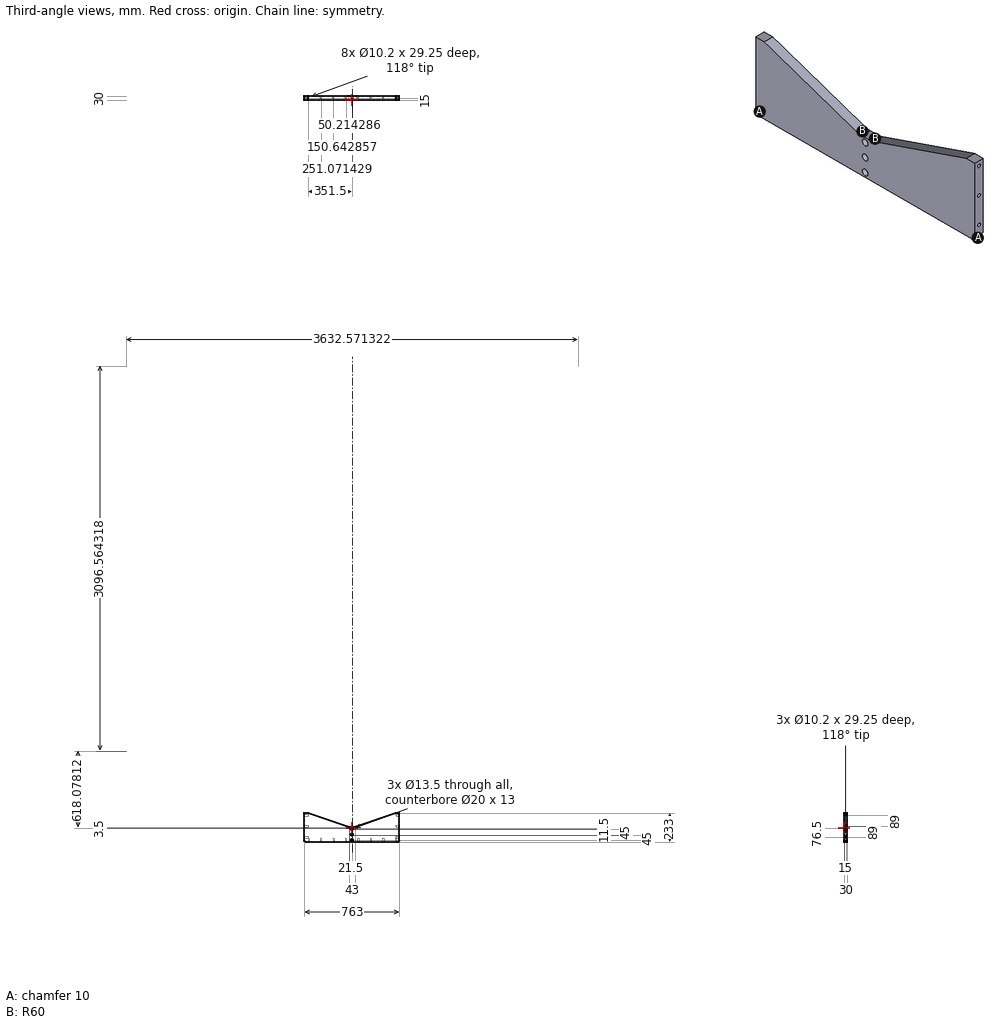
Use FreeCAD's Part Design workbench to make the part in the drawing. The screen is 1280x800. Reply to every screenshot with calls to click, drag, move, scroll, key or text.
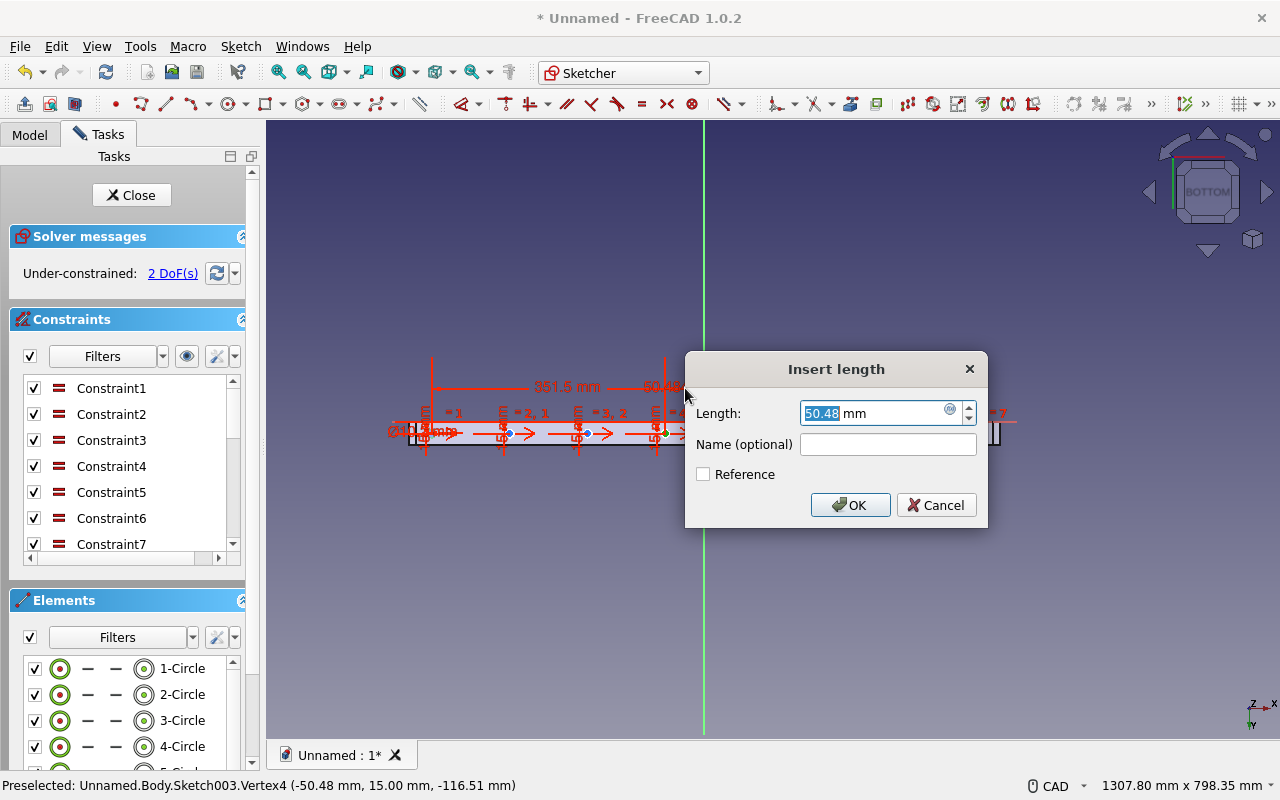
text(50.214286)
key(Return)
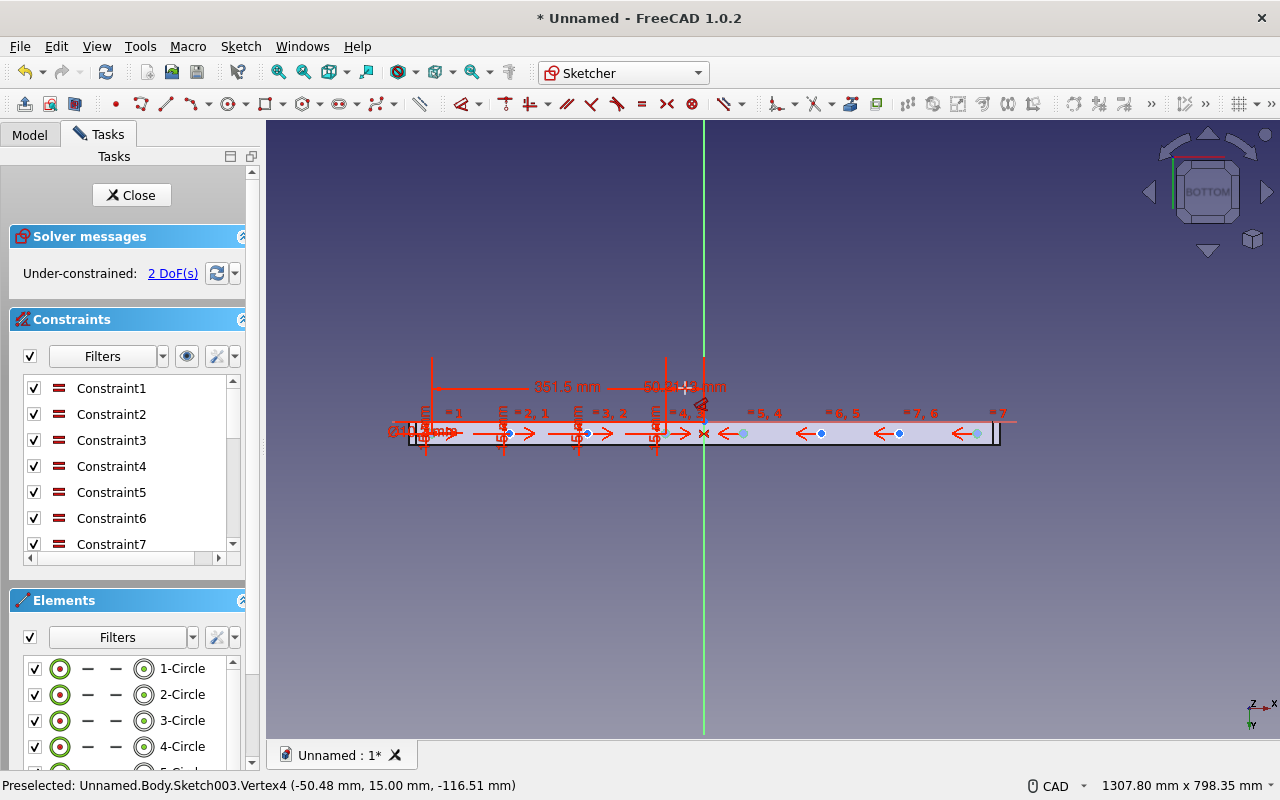
click(510, 434)
click(607, 468)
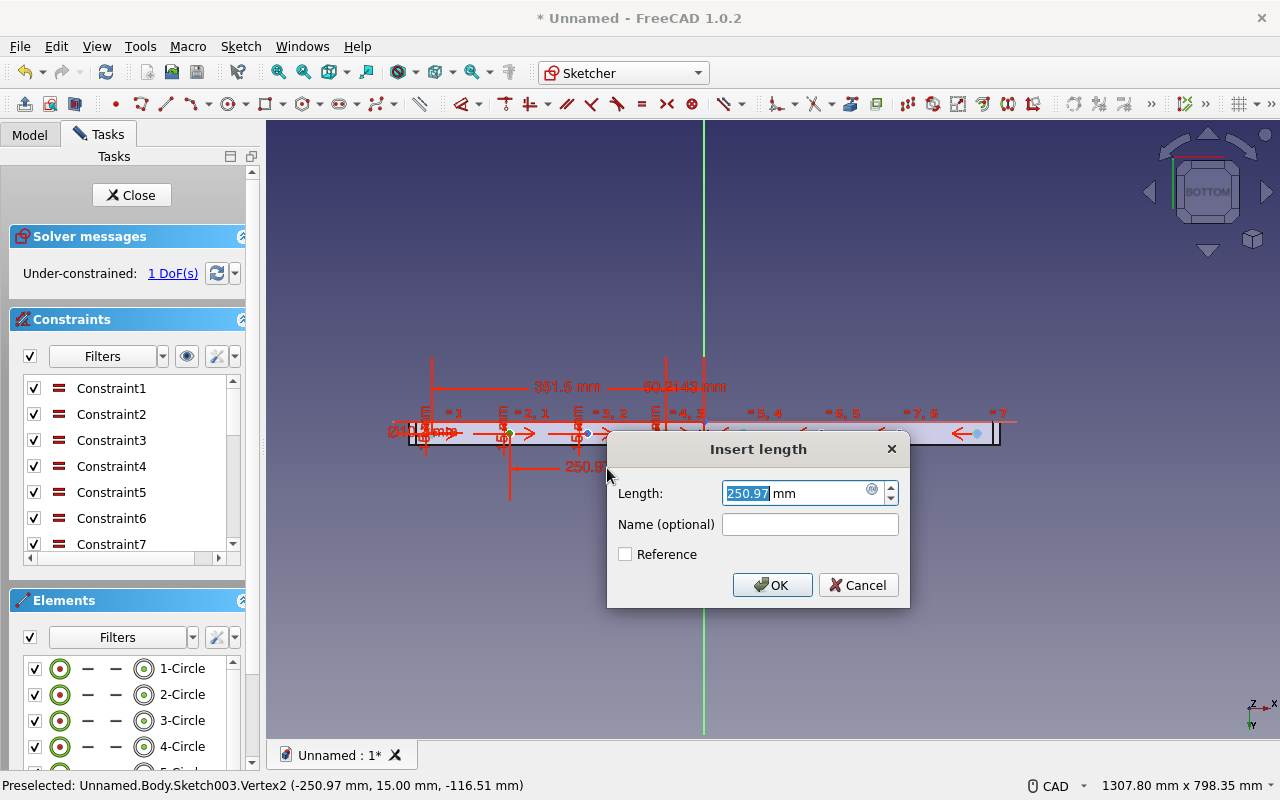
text(251.071429)
key(Return)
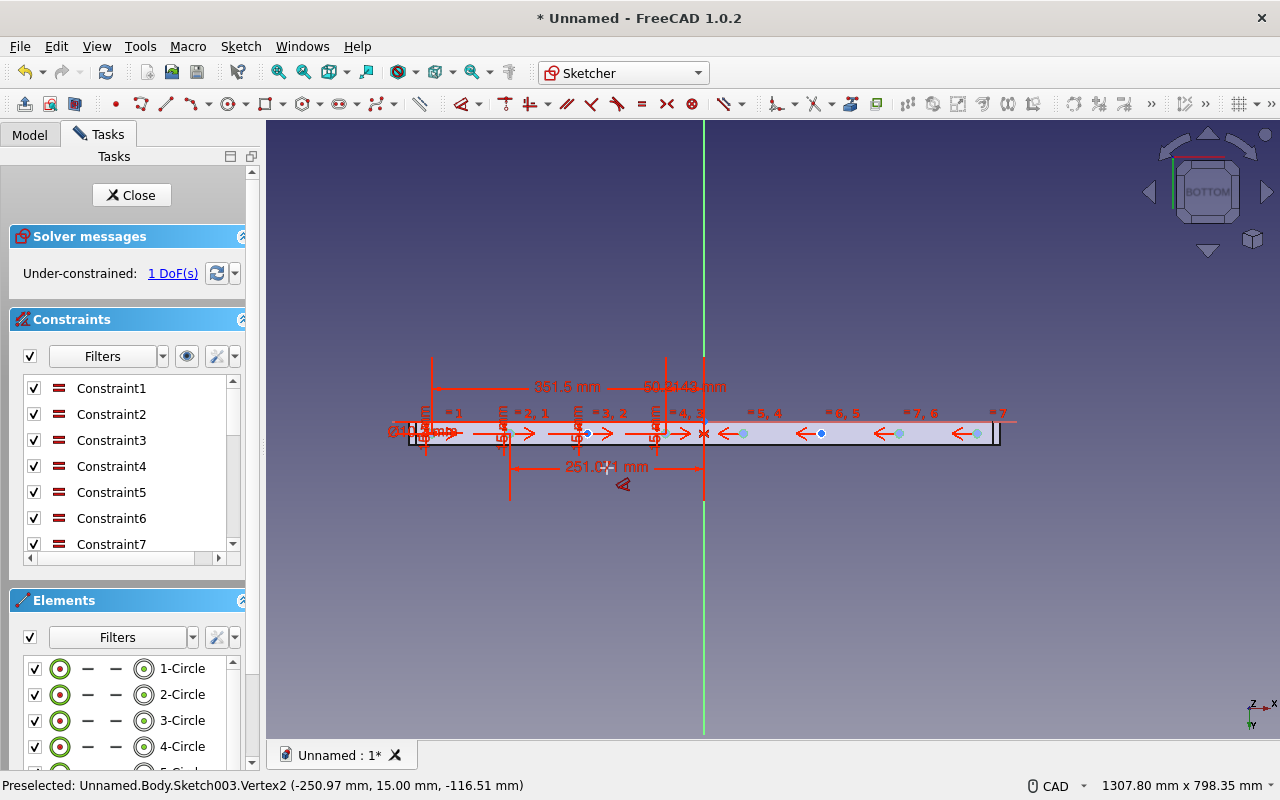
click(588, 434)
click(687, 468)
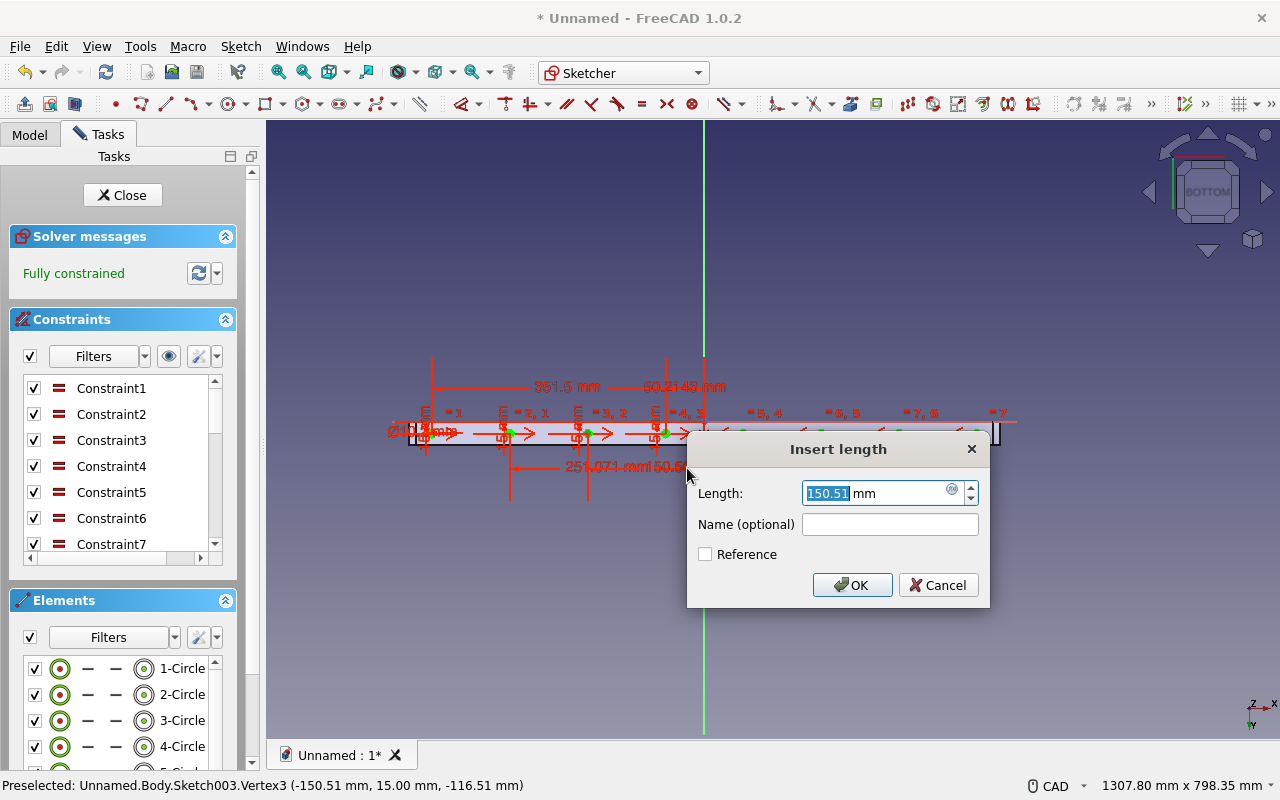
text(150.642857)
key(Return)
key(Escape)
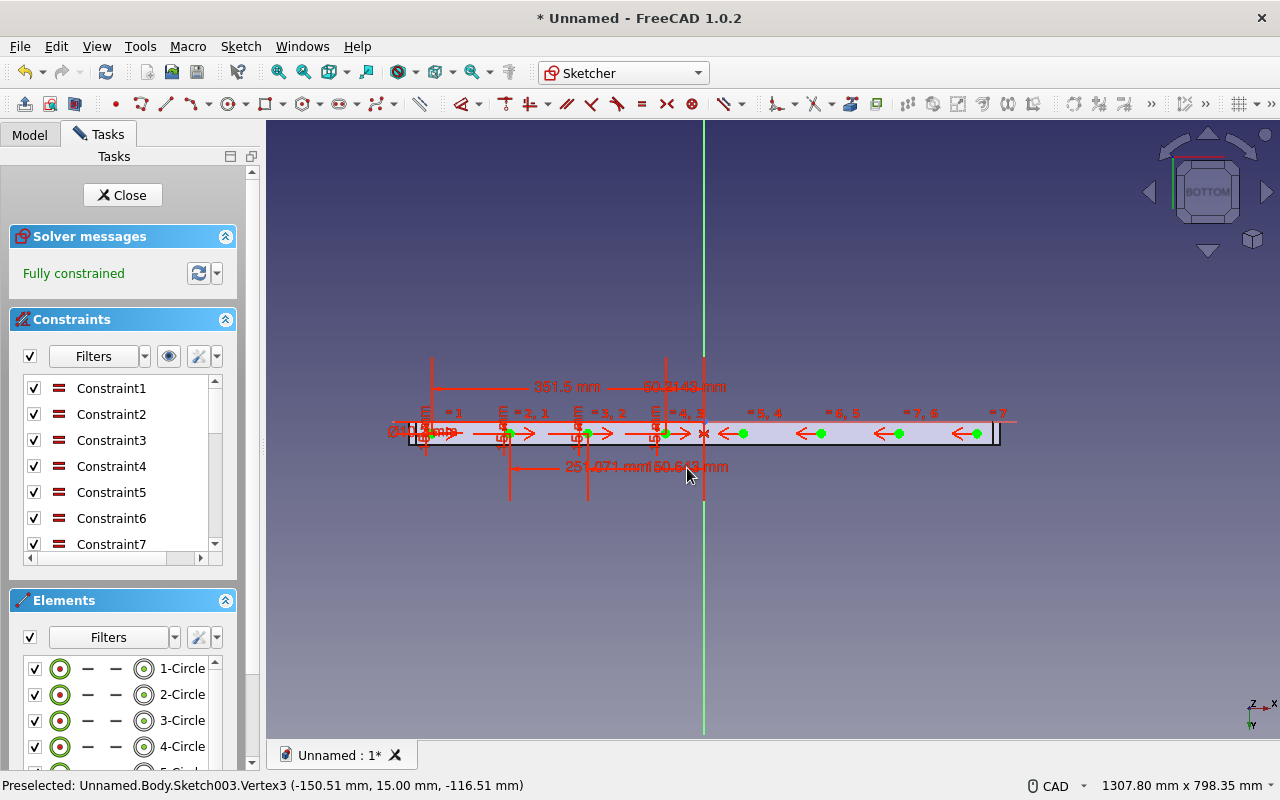
click(123, 195)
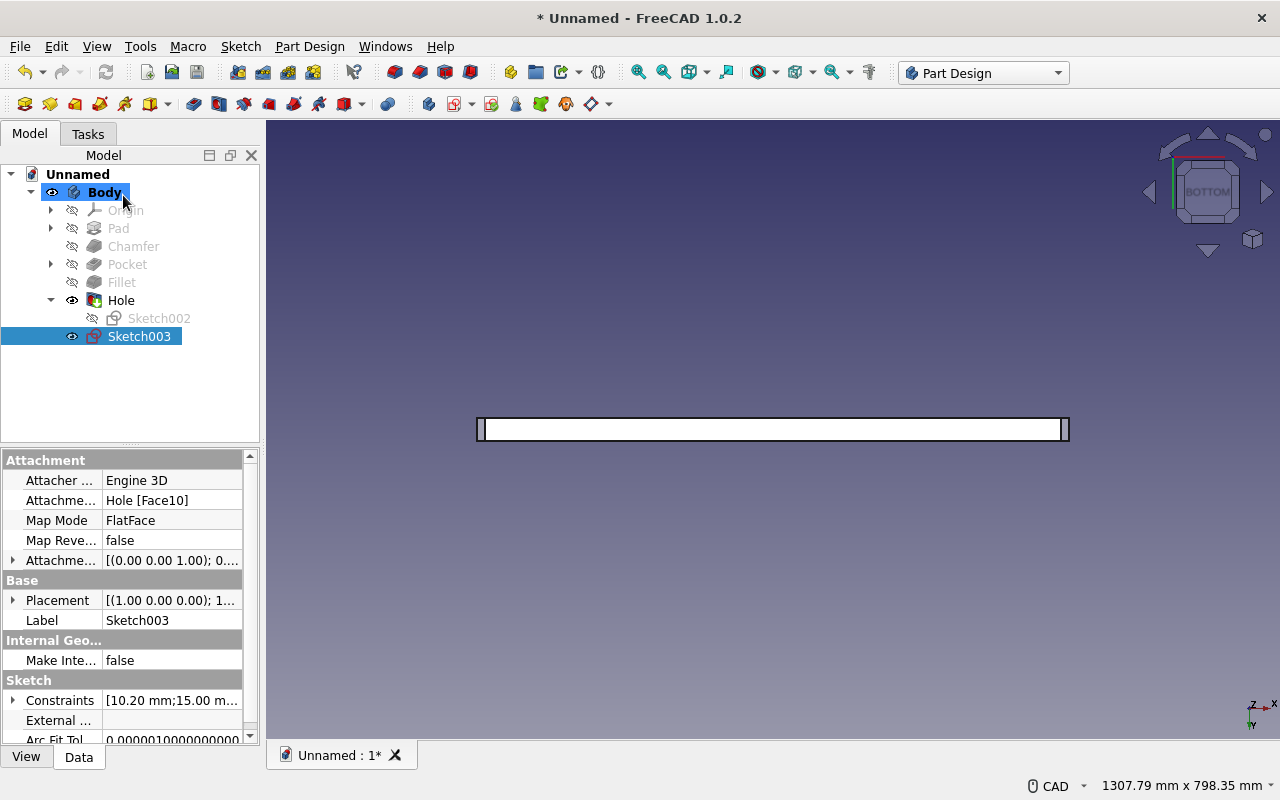
click(219, 104)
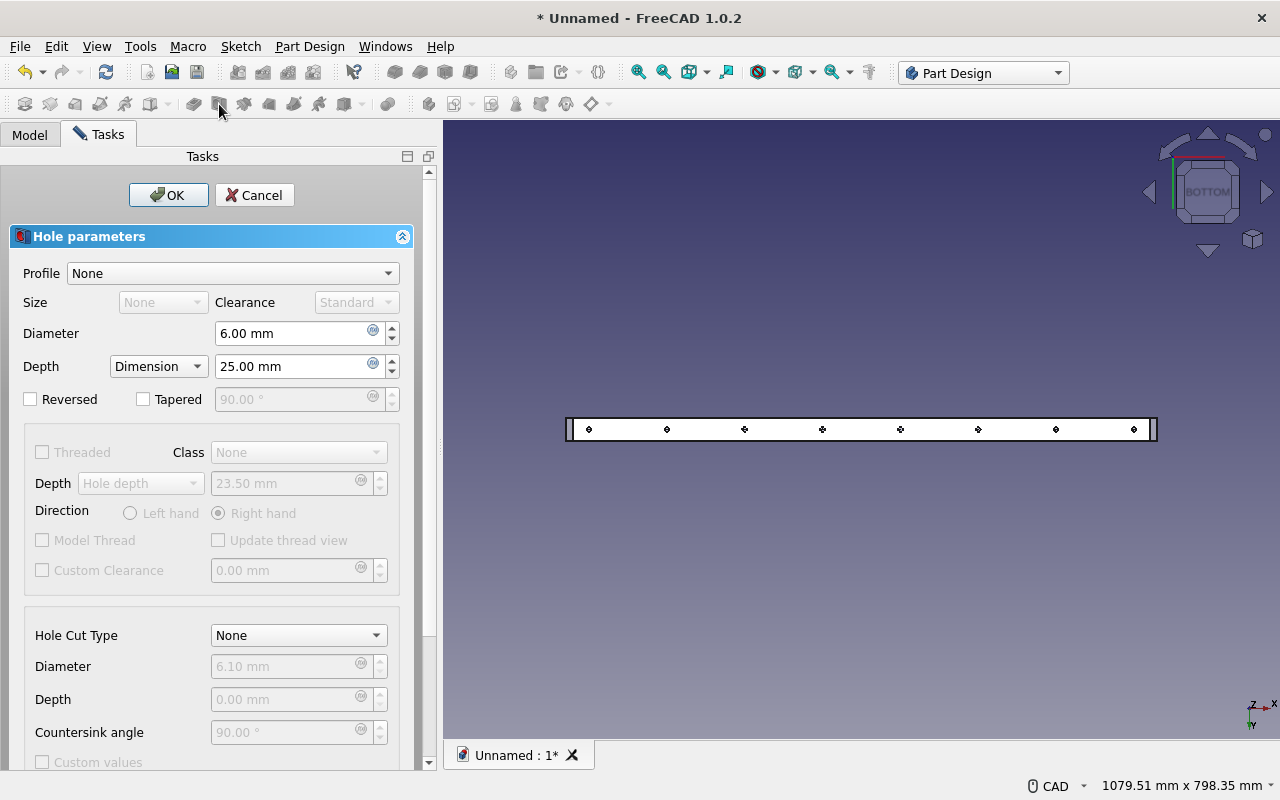
triple_click(300, 334)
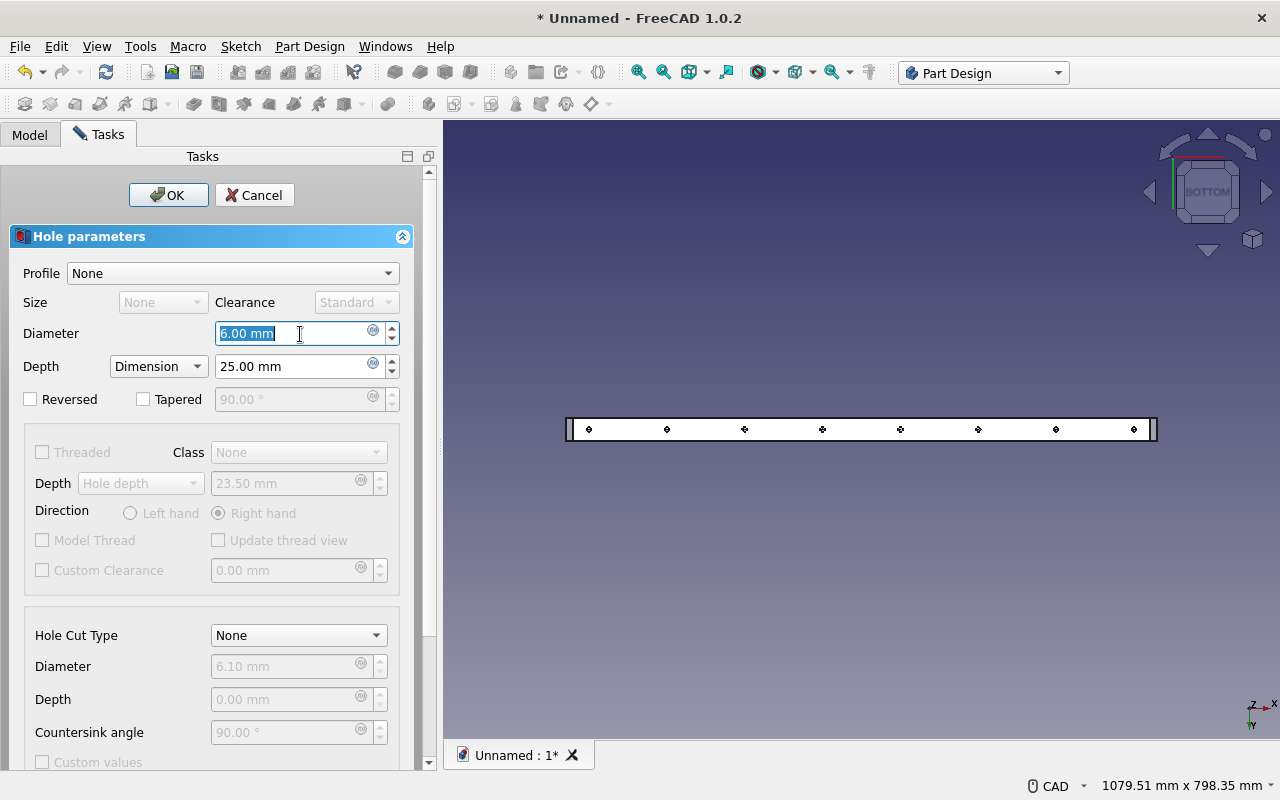
text(10.2)
key(Tab)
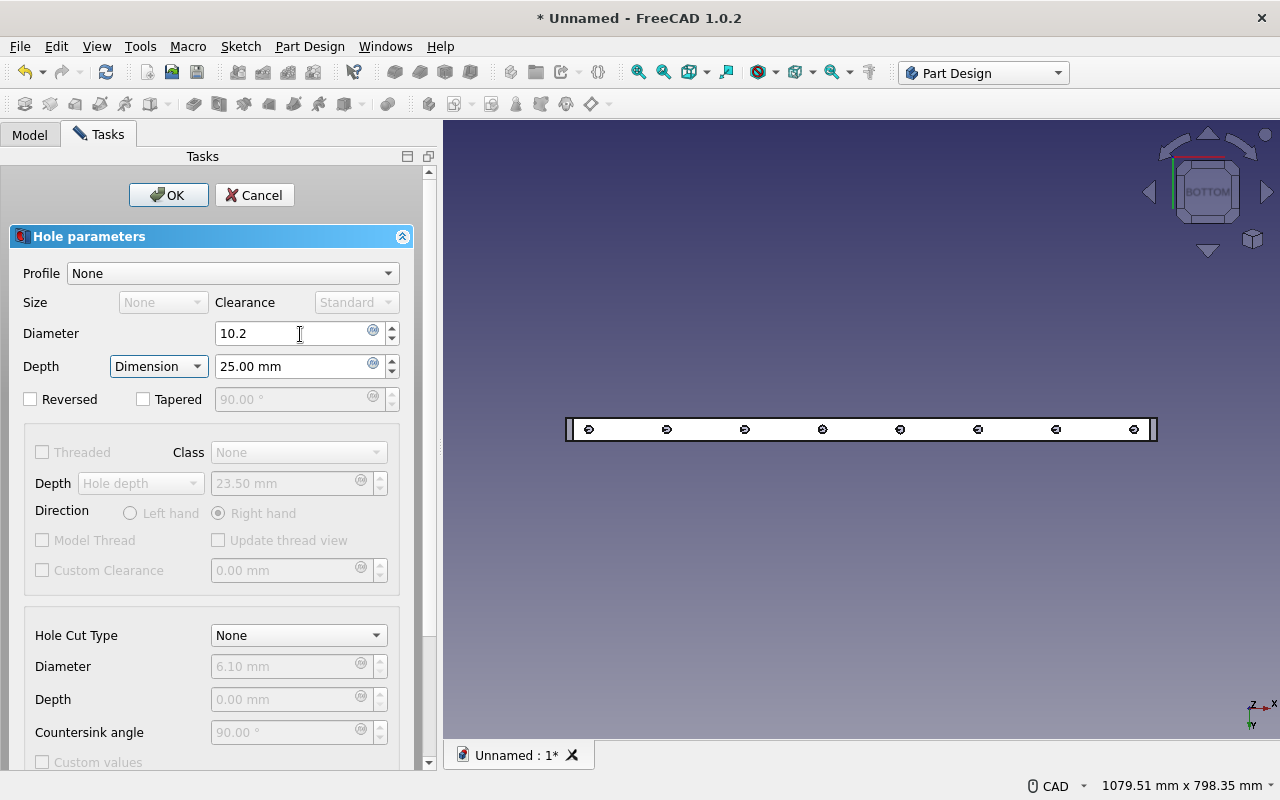
triple_click(300, 366)